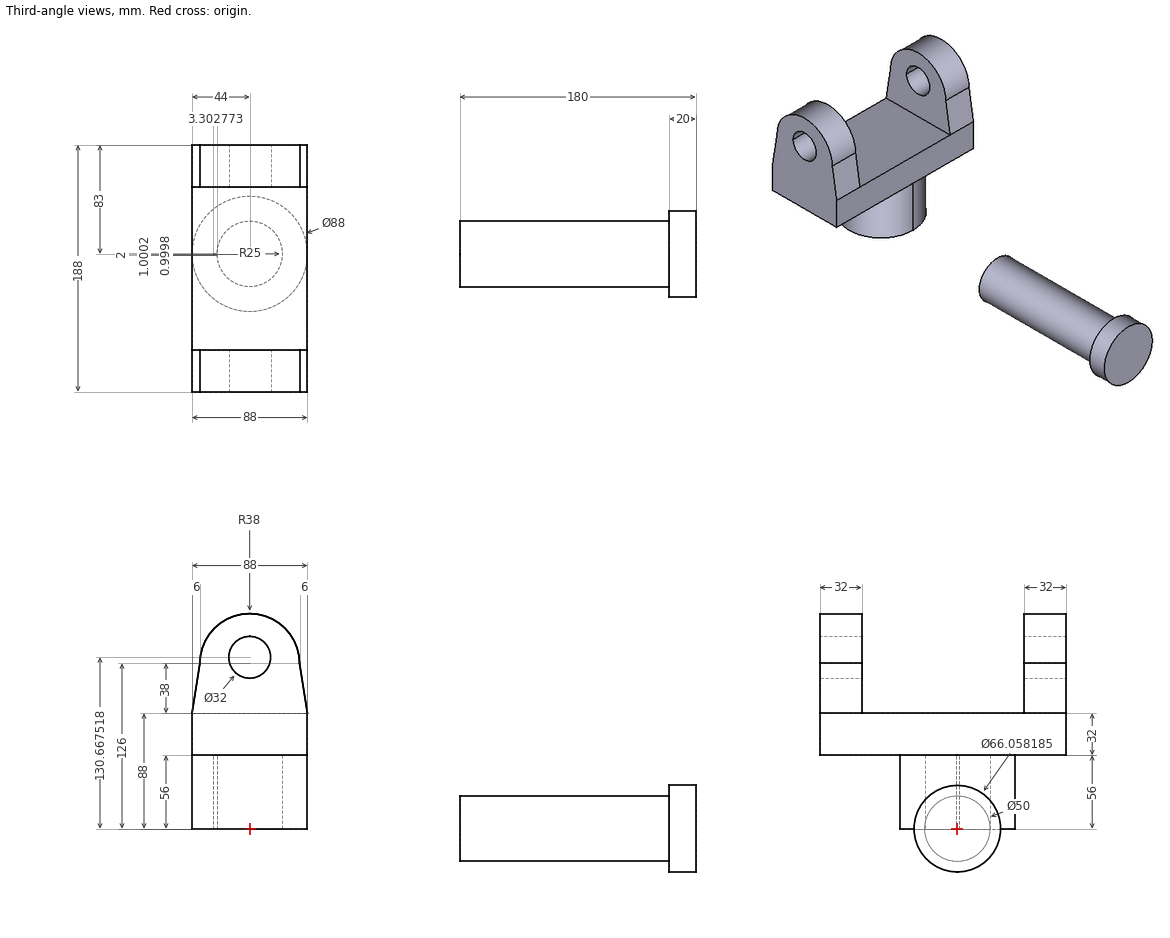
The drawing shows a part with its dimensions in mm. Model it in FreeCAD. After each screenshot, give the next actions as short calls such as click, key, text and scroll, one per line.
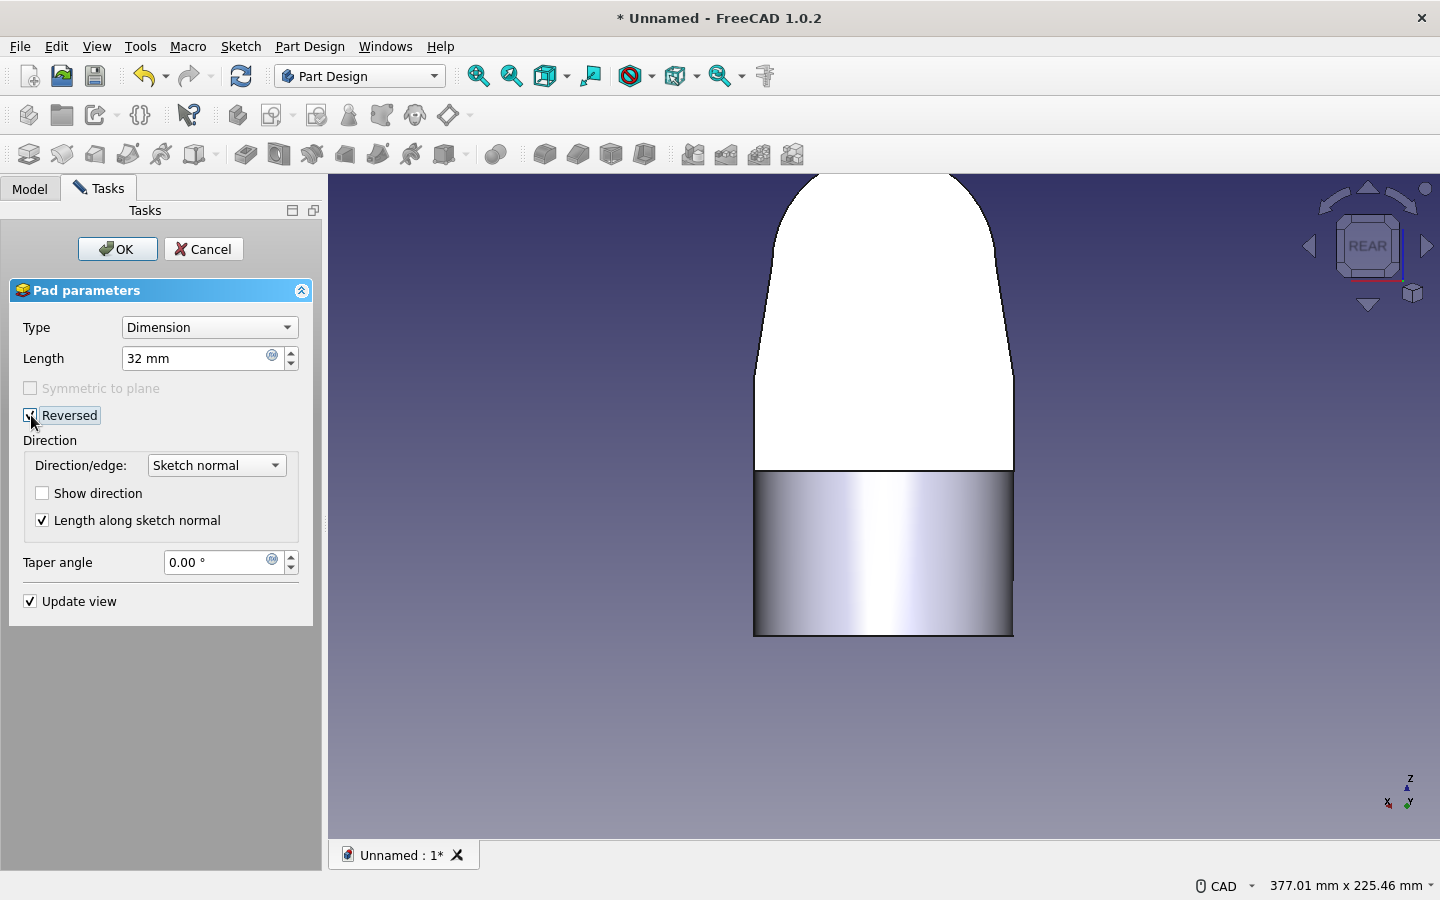
click(118, 249)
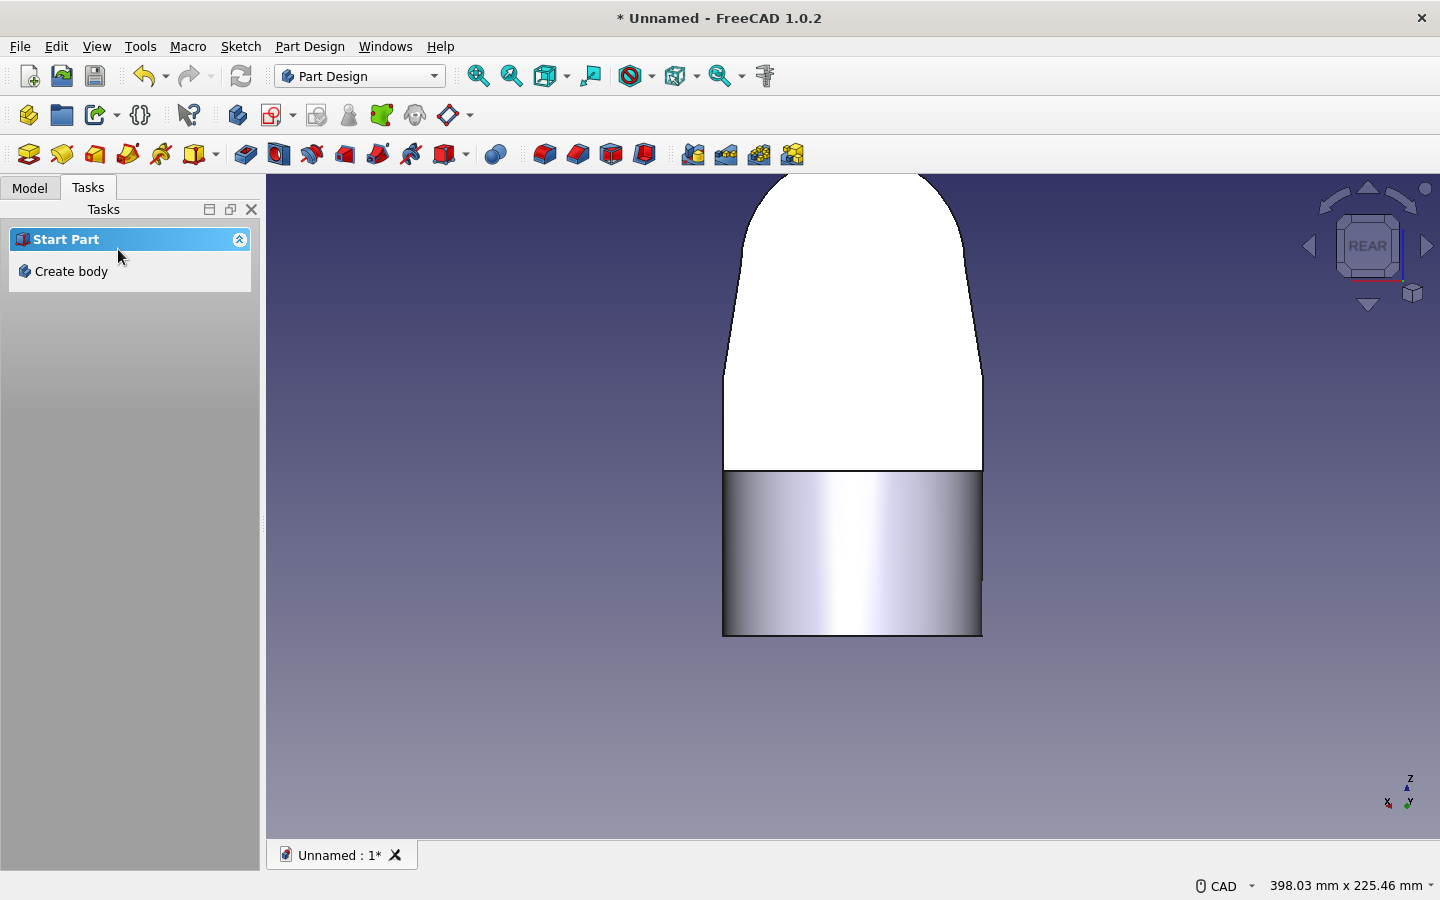
click(479, 76)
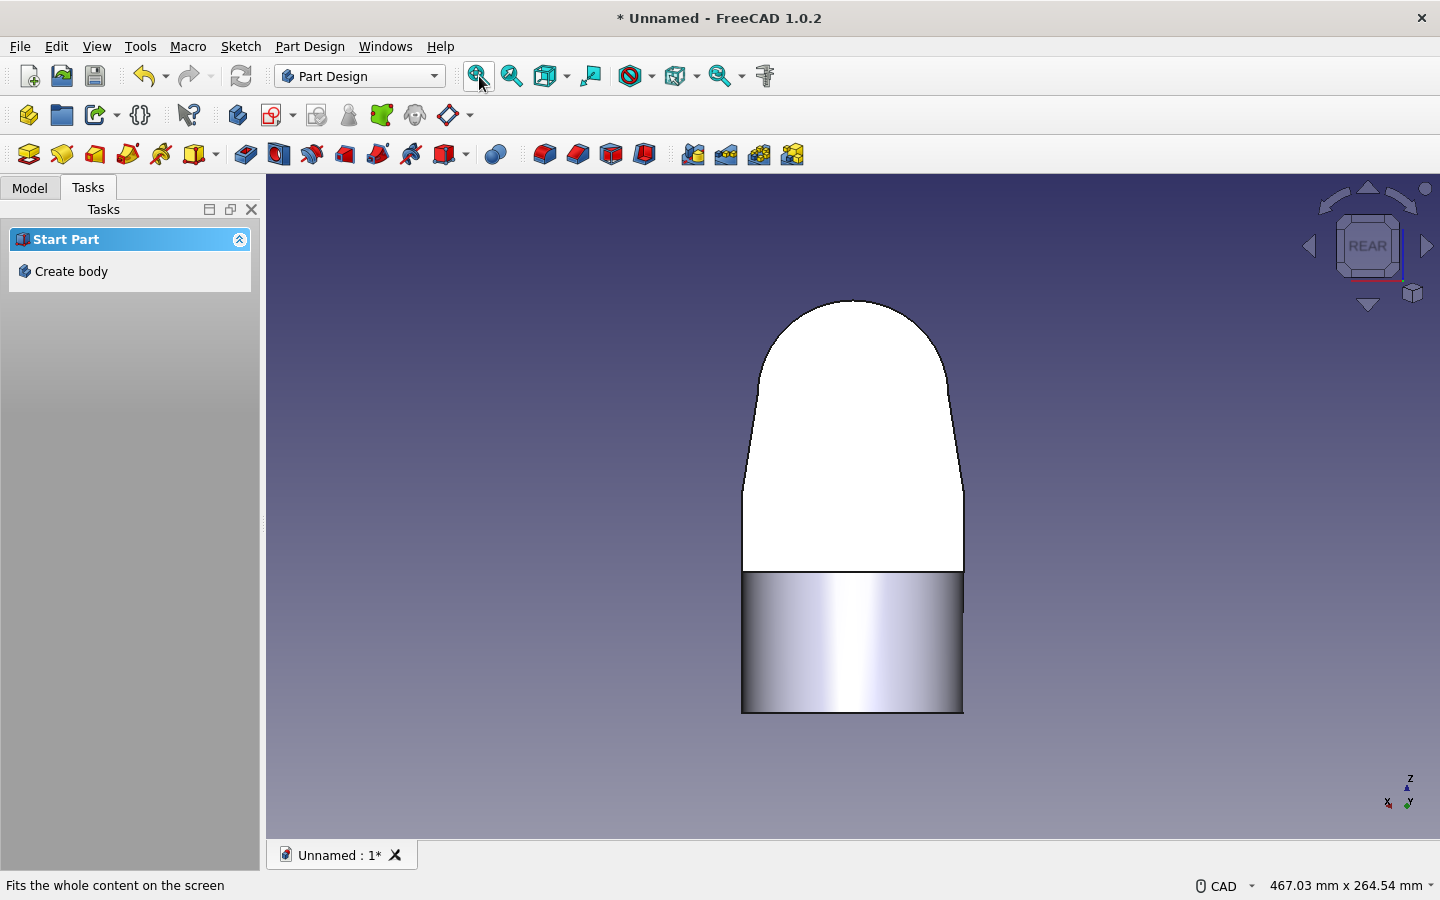
click(30, 188)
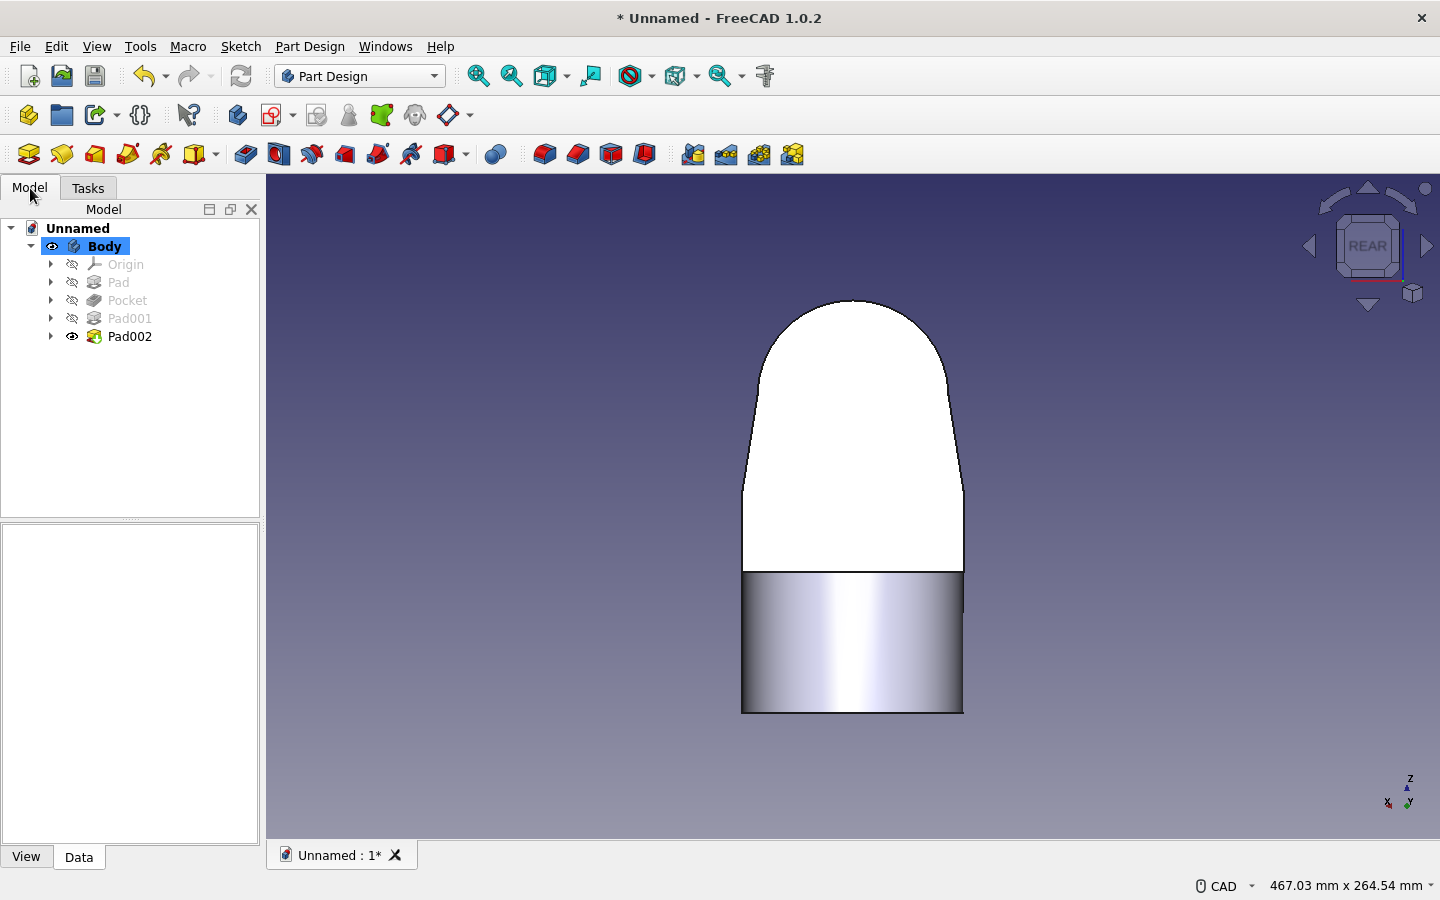
click(51, 264)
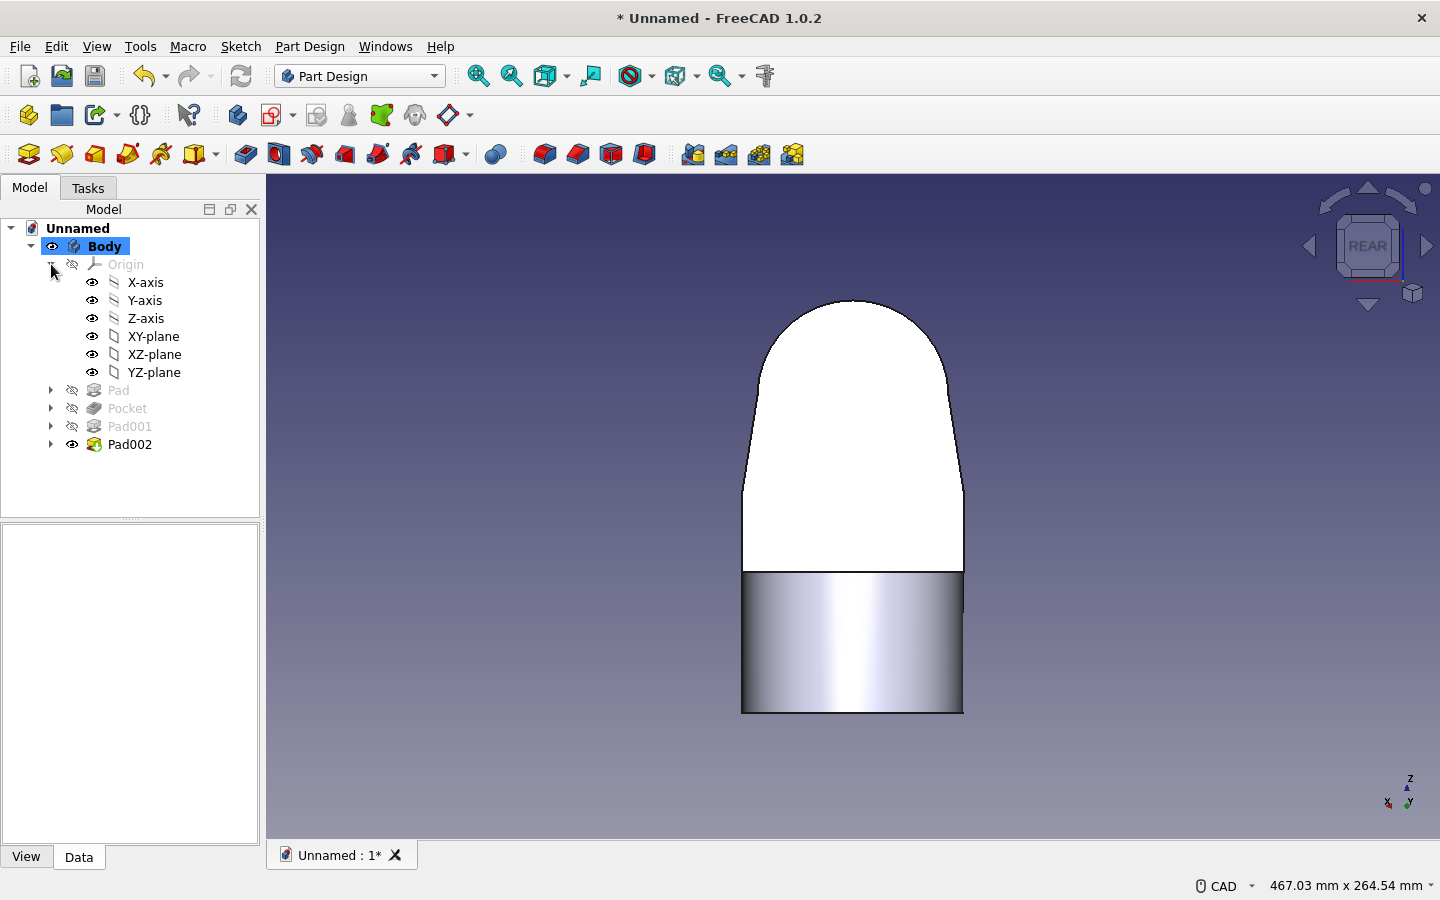
click(137, 354)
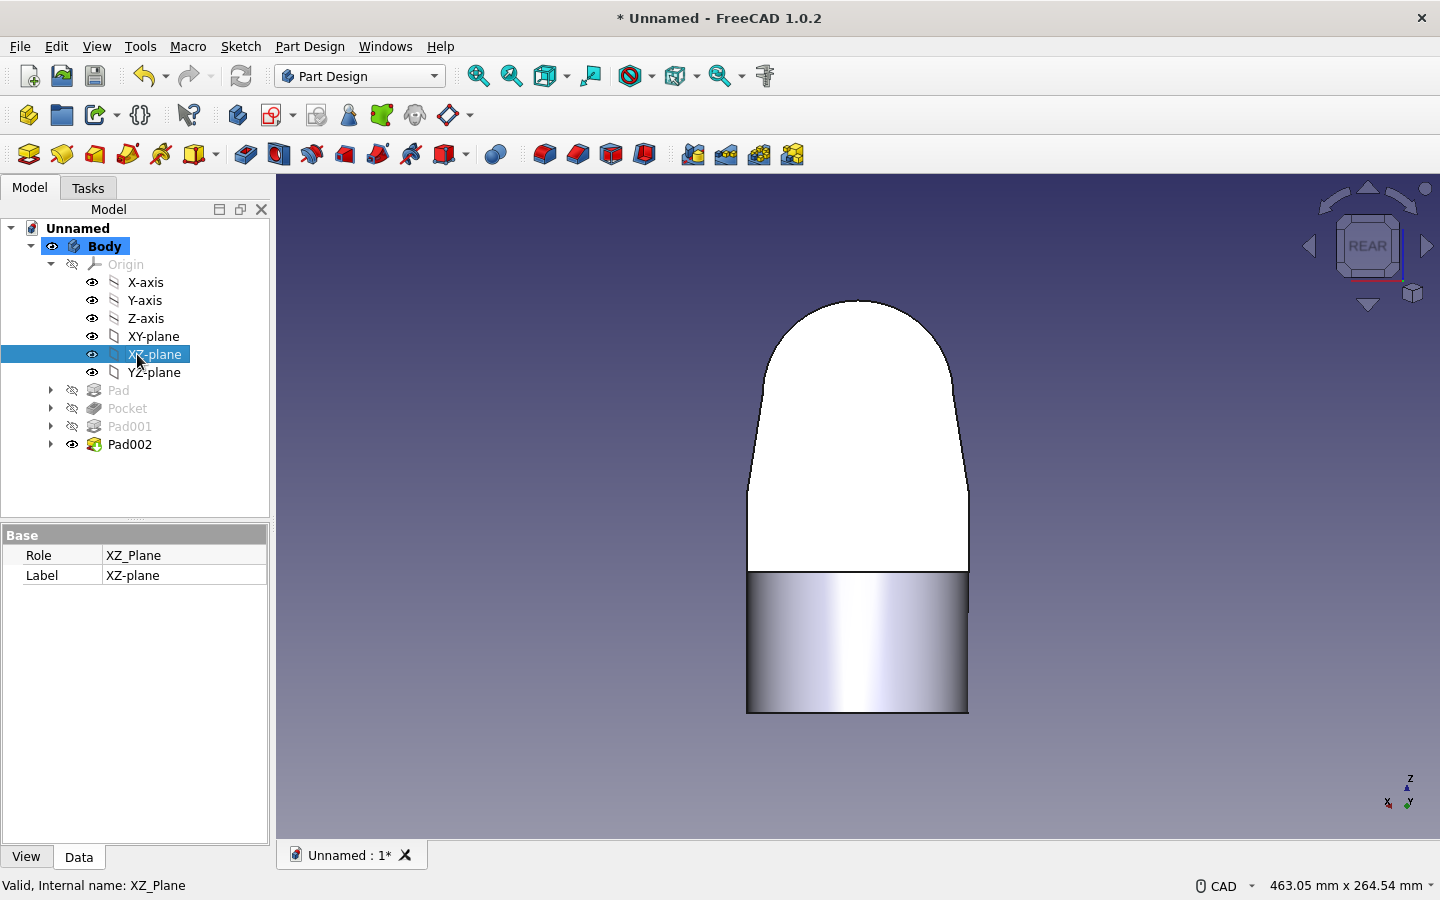
click(448, 116)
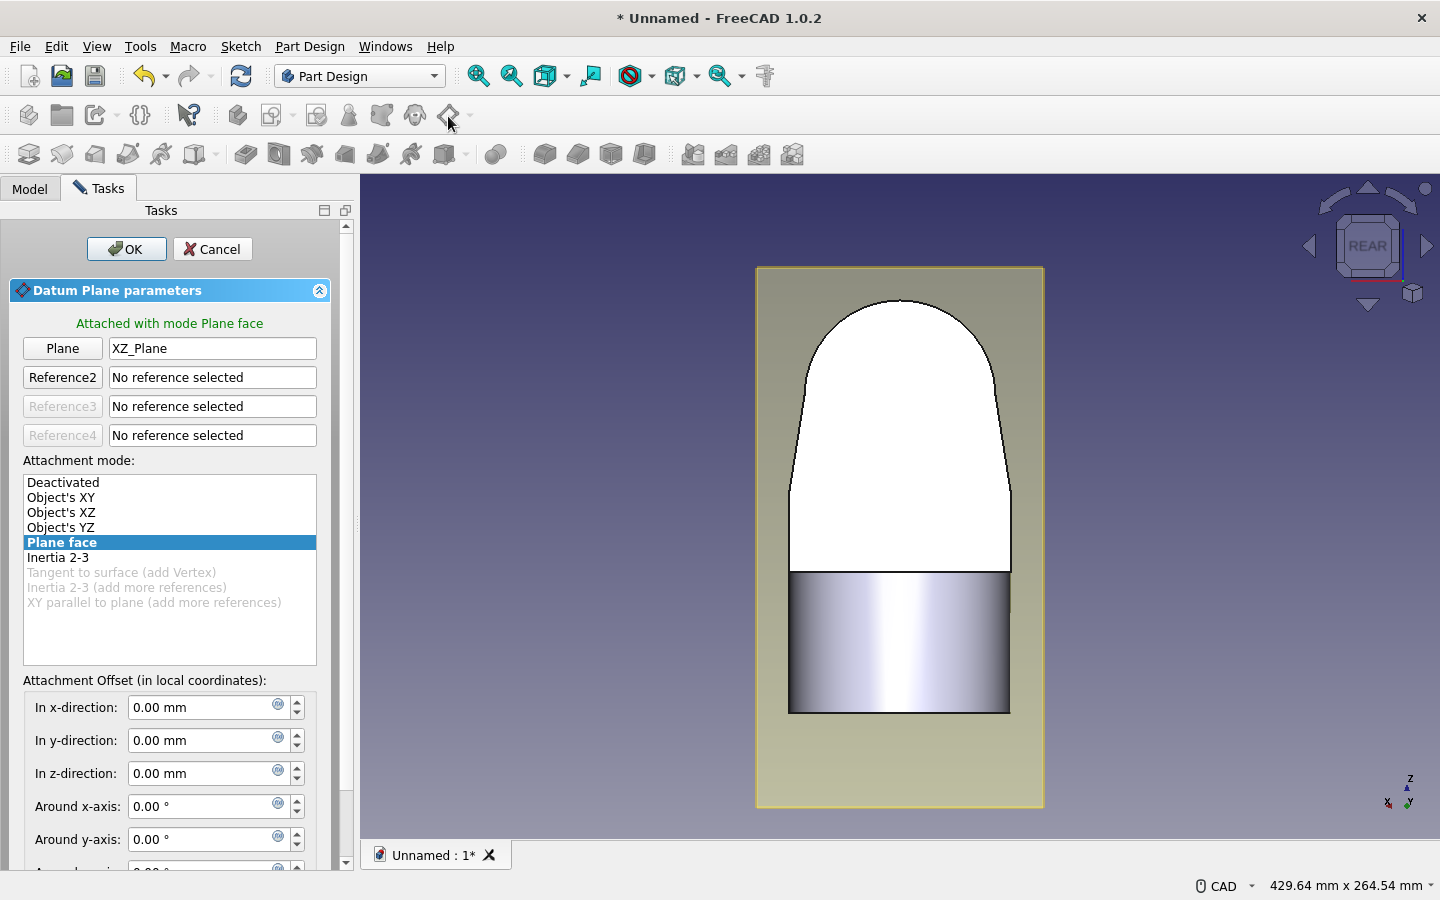
triple_click(210, 774)